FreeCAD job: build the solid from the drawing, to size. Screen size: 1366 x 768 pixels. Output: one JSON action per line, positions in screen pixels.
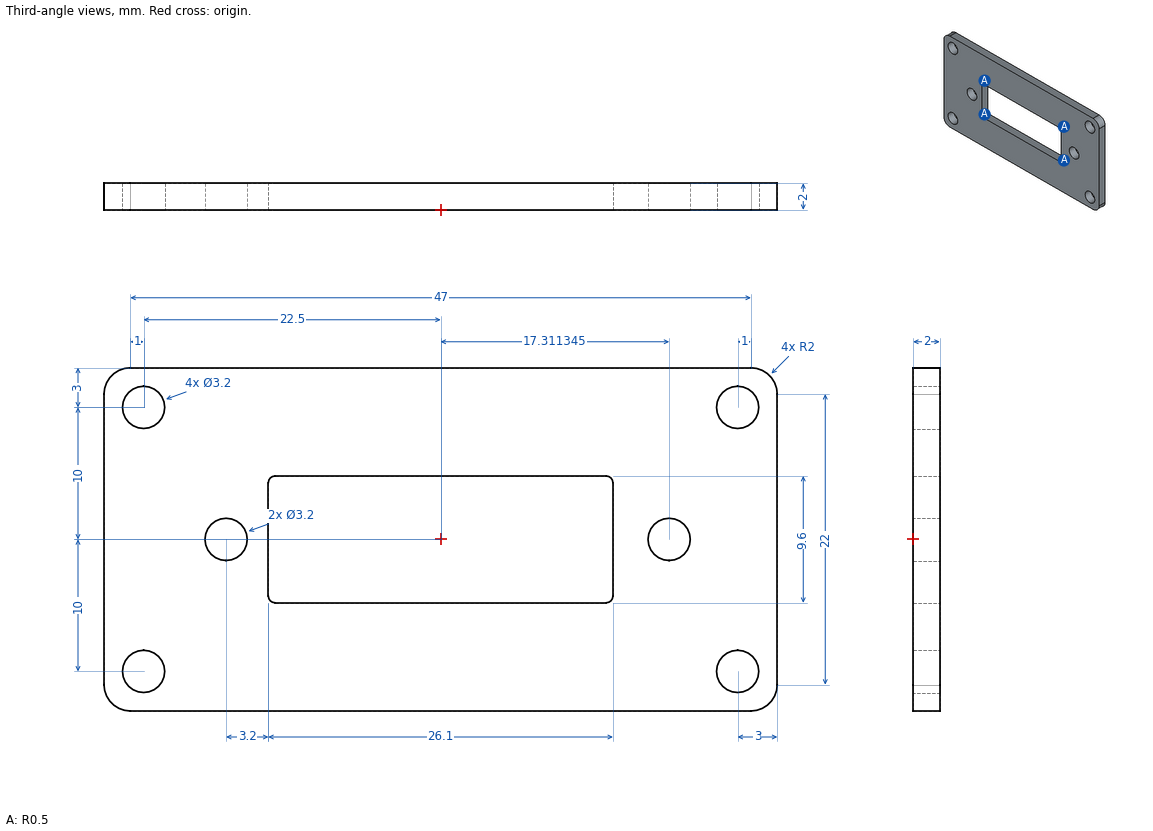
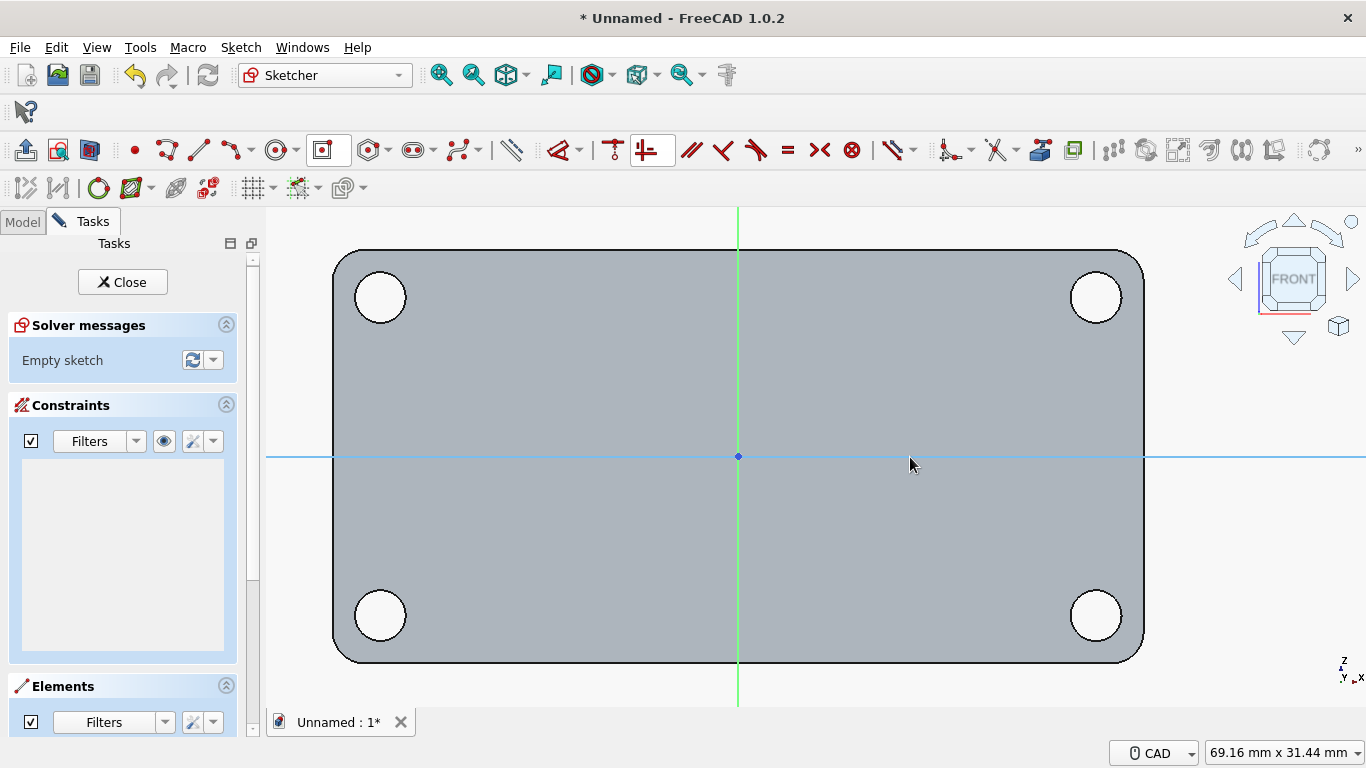
{"action": "left_click", "coordinate": [322, 150]}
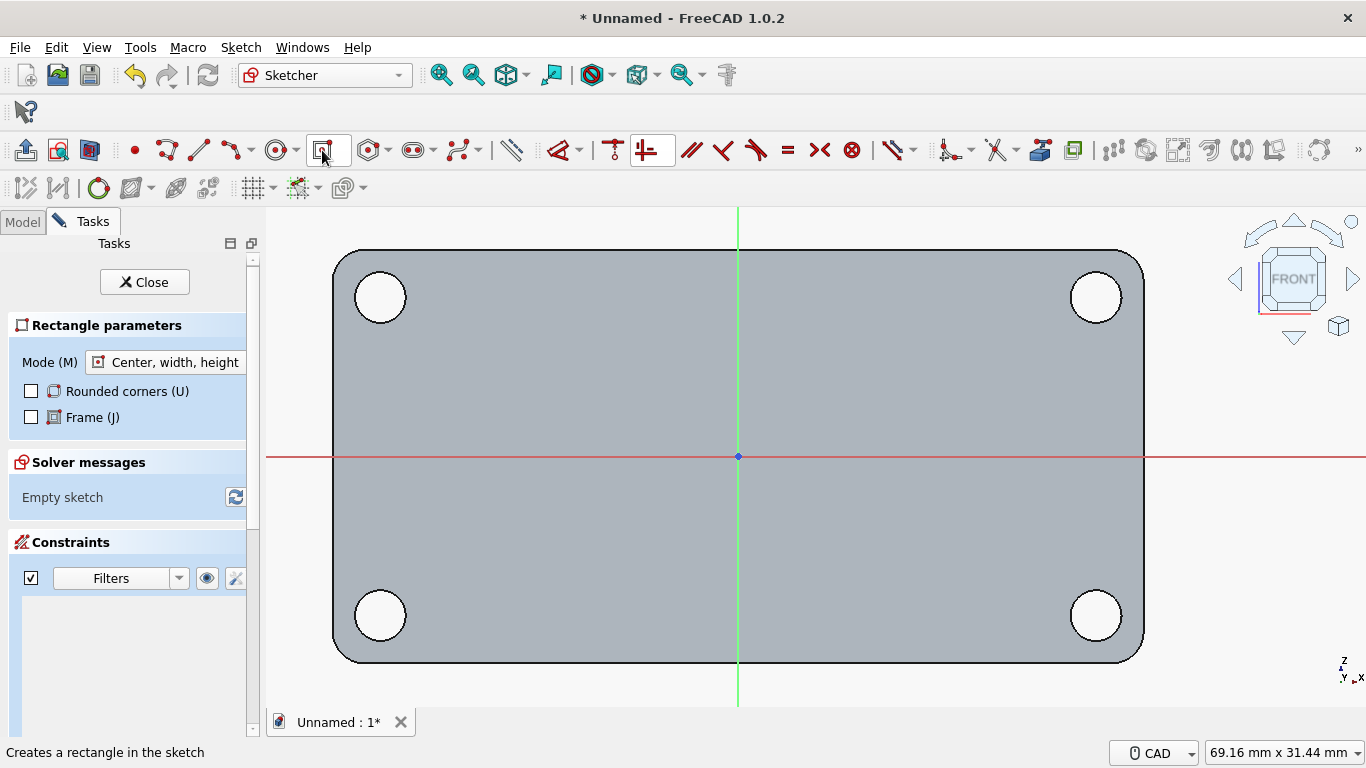
{"action": "left_click", "coordinate": [738, 457]}
{"action": "left_click", "coordinate": [946, 380]}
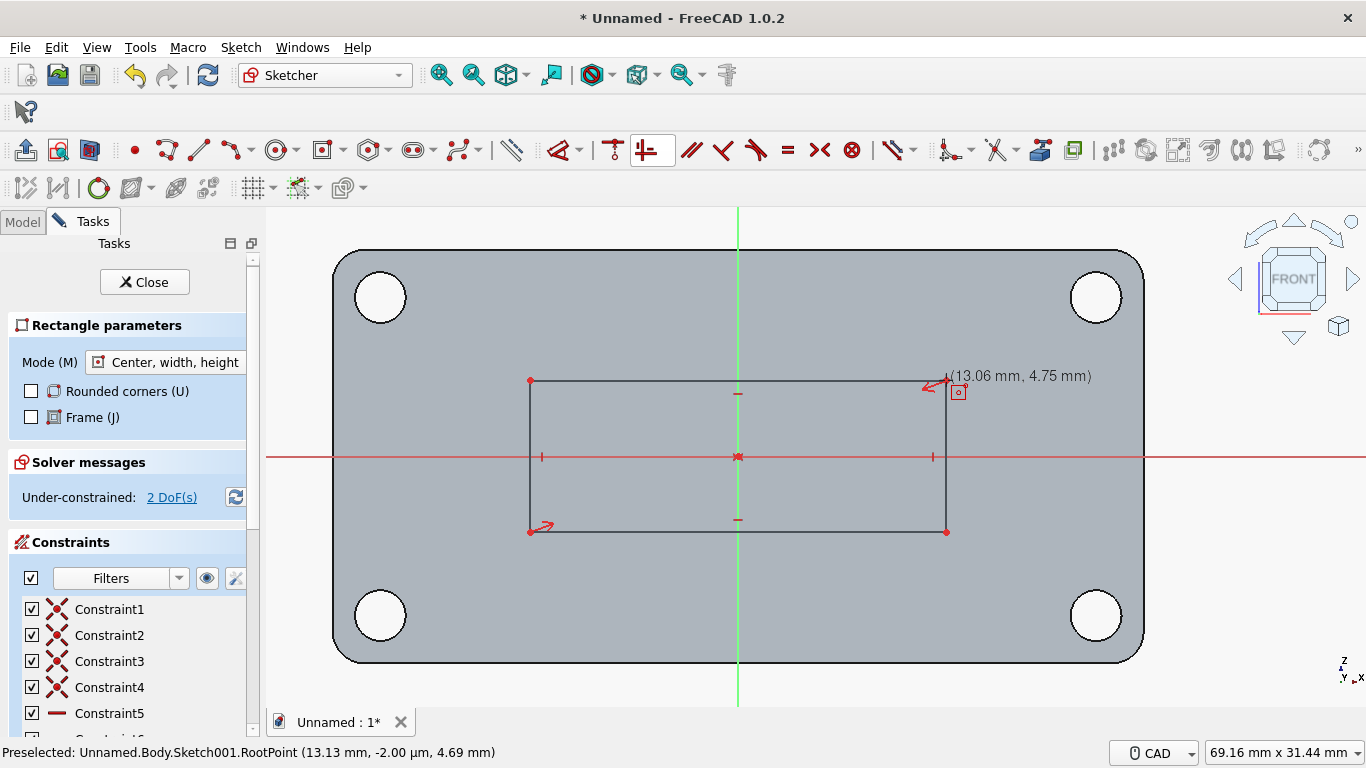
{"action": "left_click", "coordinate": [276, 150]}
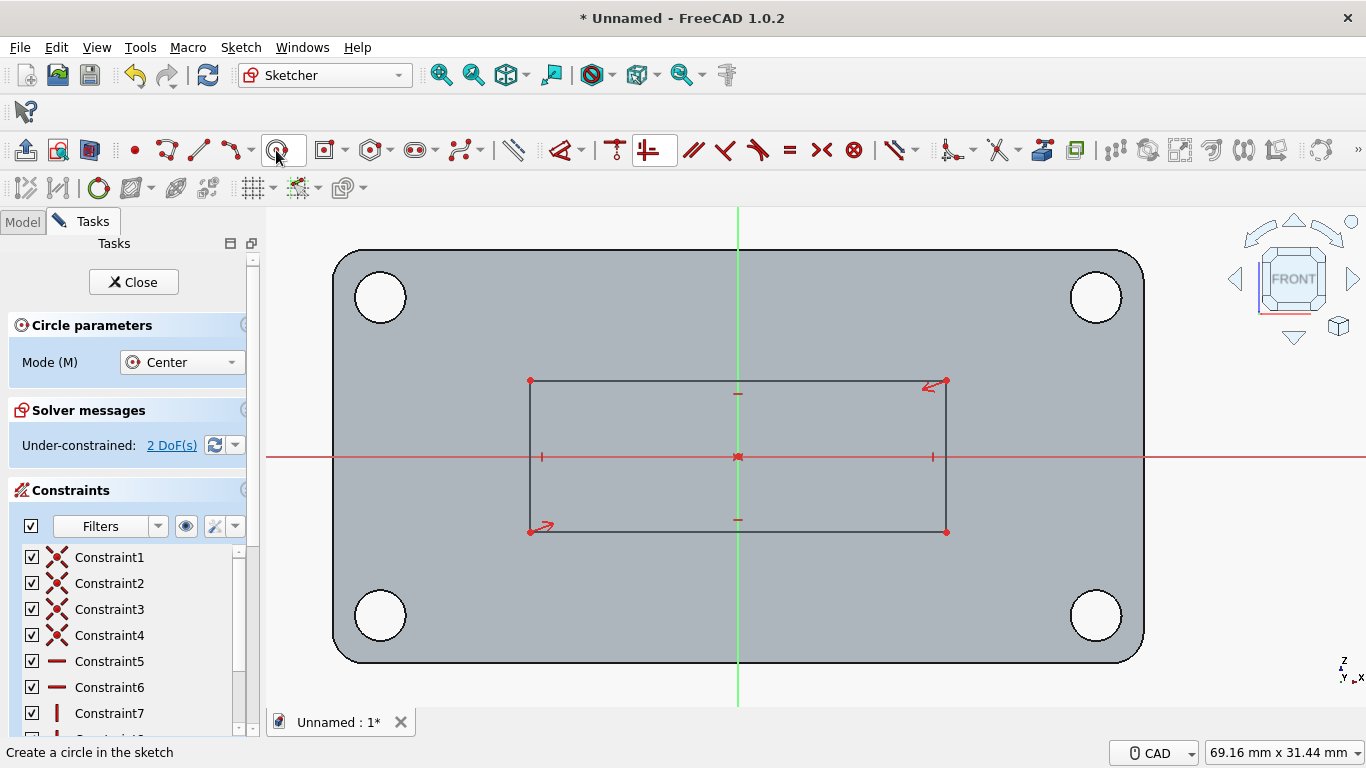
{"action": "left_click", "coordinate": [480, 457]}
{"action": "left_click", "coordinate": [498, 439]}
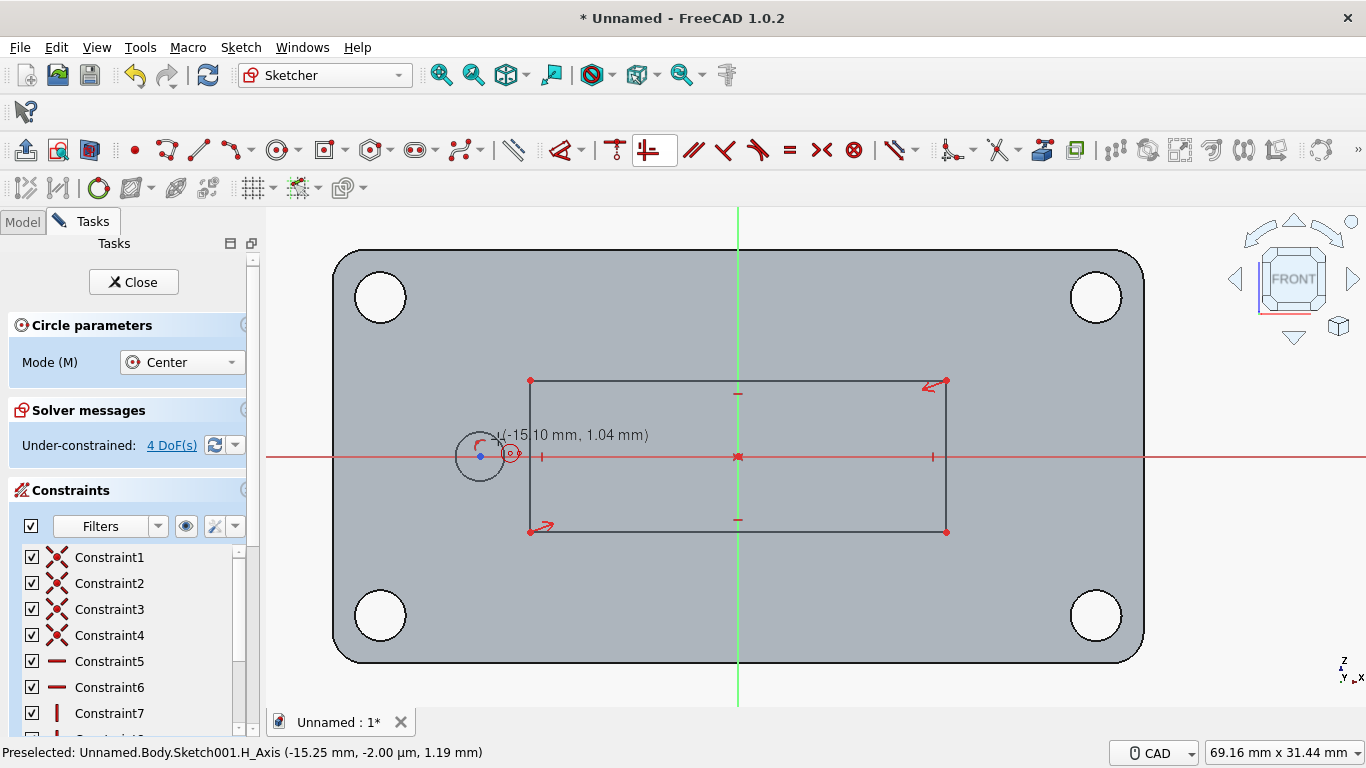
{"action": "left_click", "coordinate": [1014, 457]}
{"action": "left_click", "coordinate": [1032, 439]}
{"action": "key", "text": "Escape"}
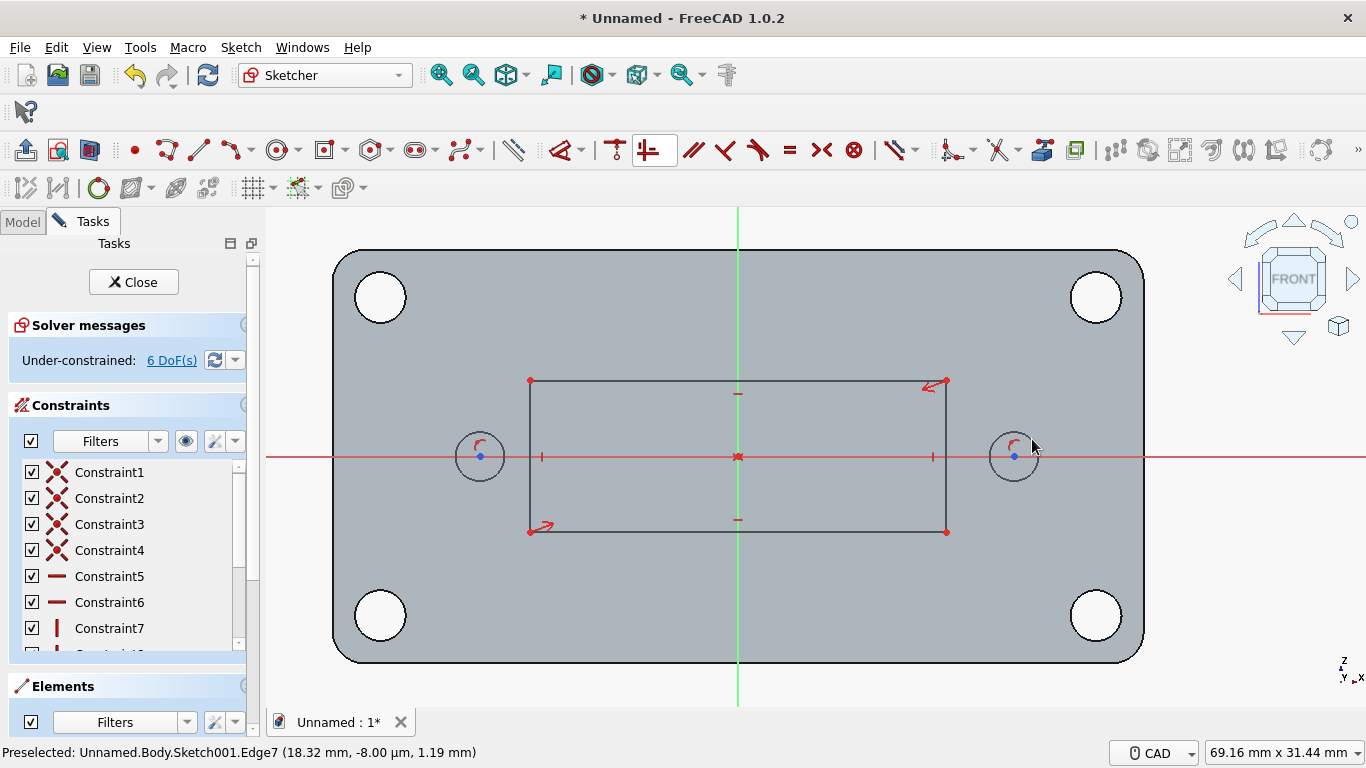
{"action": "left_click", "coordinate": [497, 439]}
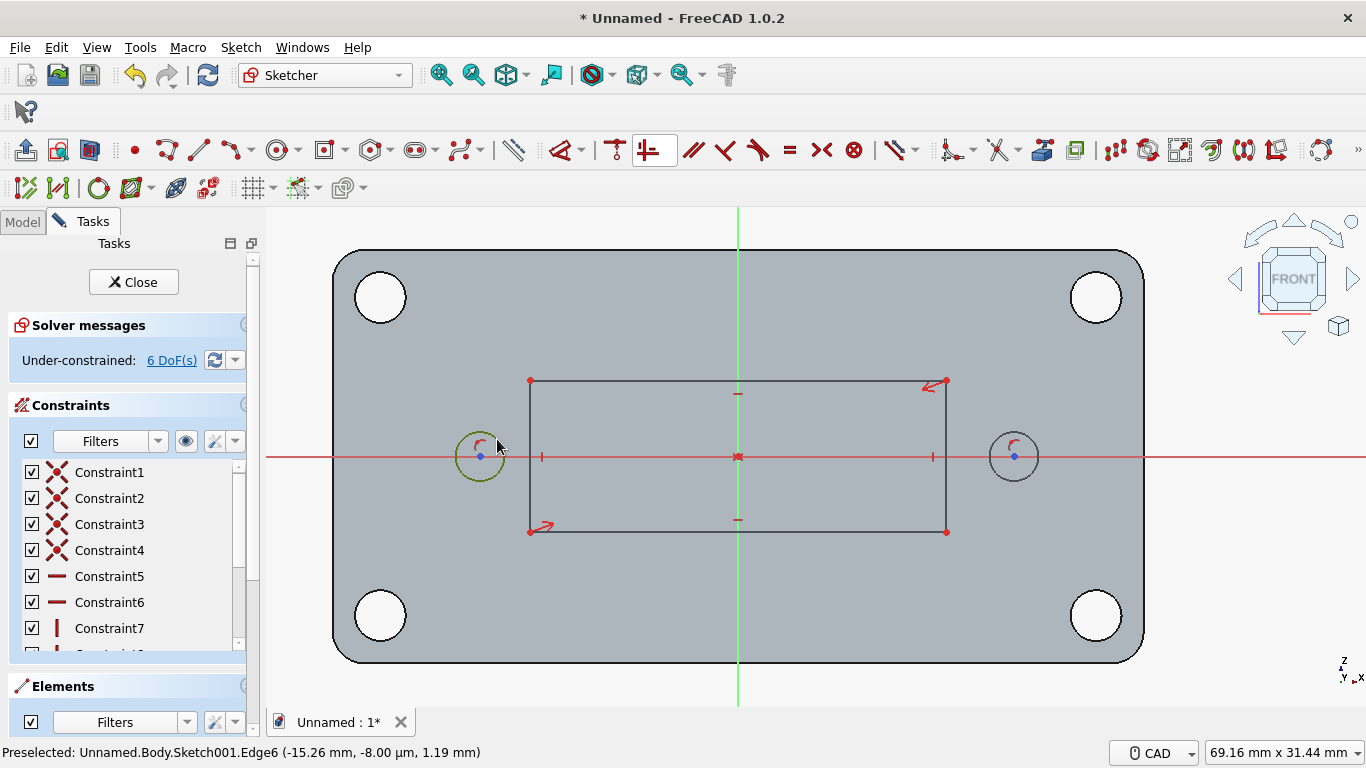
{"action": "left_click", "coordinate": [1031, 439]}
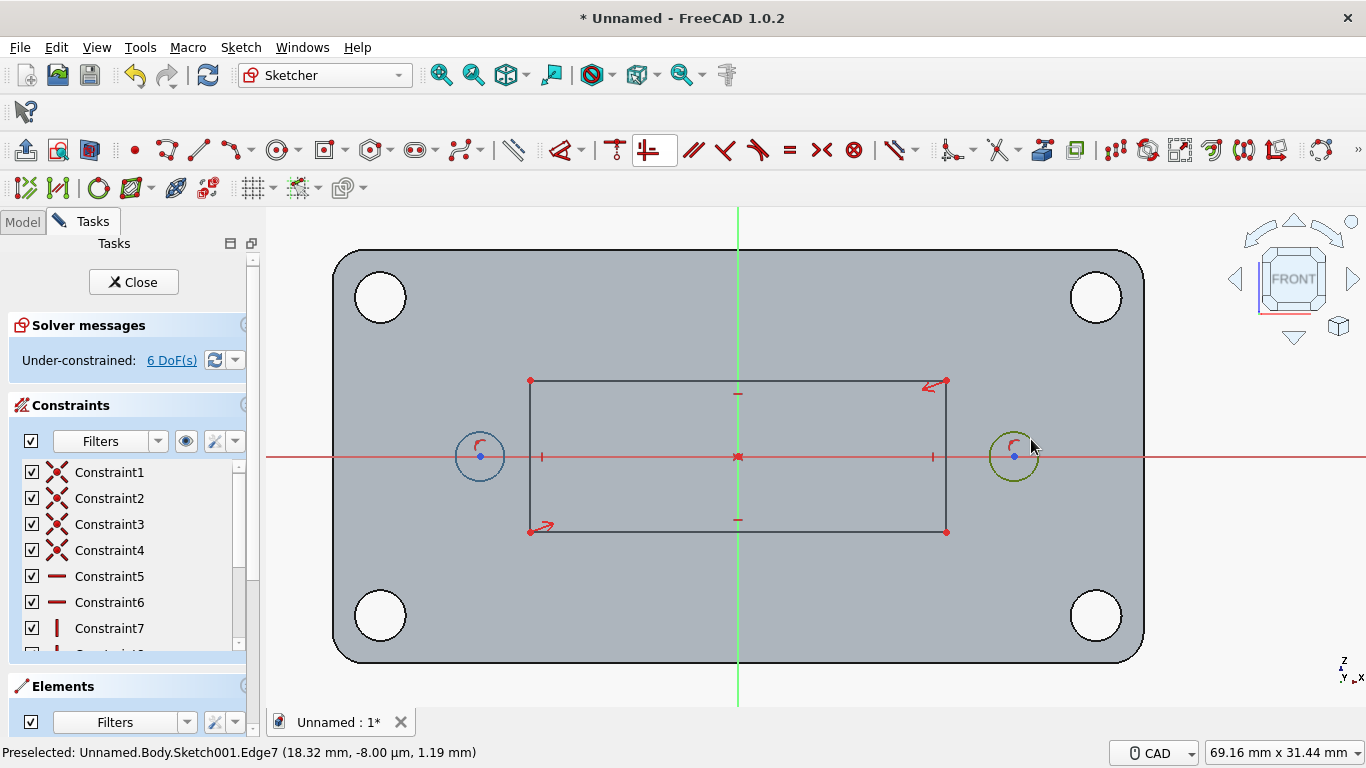
{"action": "left_click", "coordinate": [790, 150]}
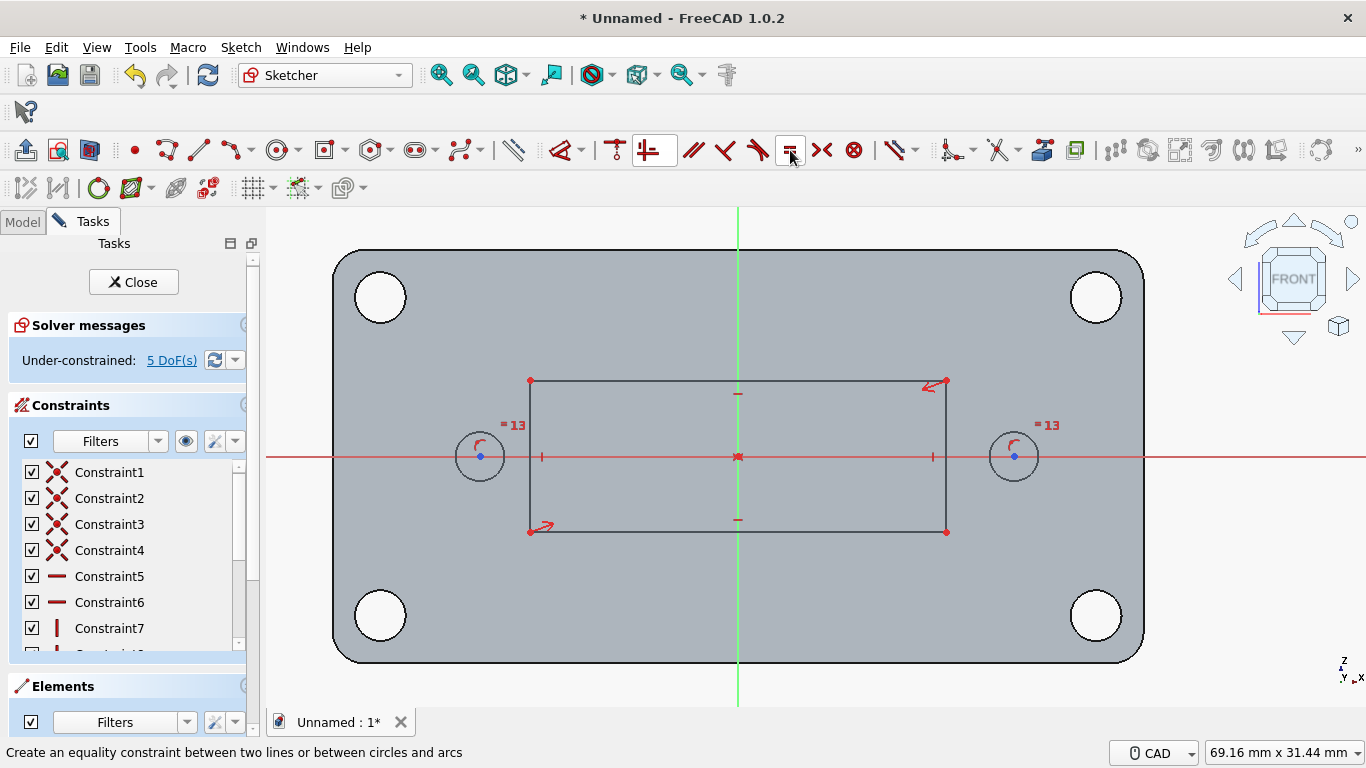
{"action": "left_click", "coordinate": [560, 150]}